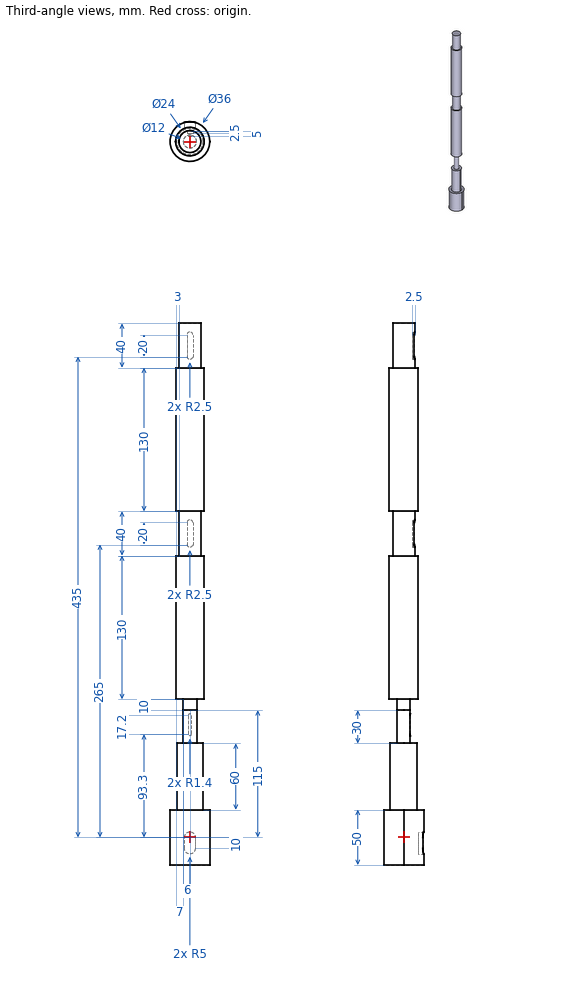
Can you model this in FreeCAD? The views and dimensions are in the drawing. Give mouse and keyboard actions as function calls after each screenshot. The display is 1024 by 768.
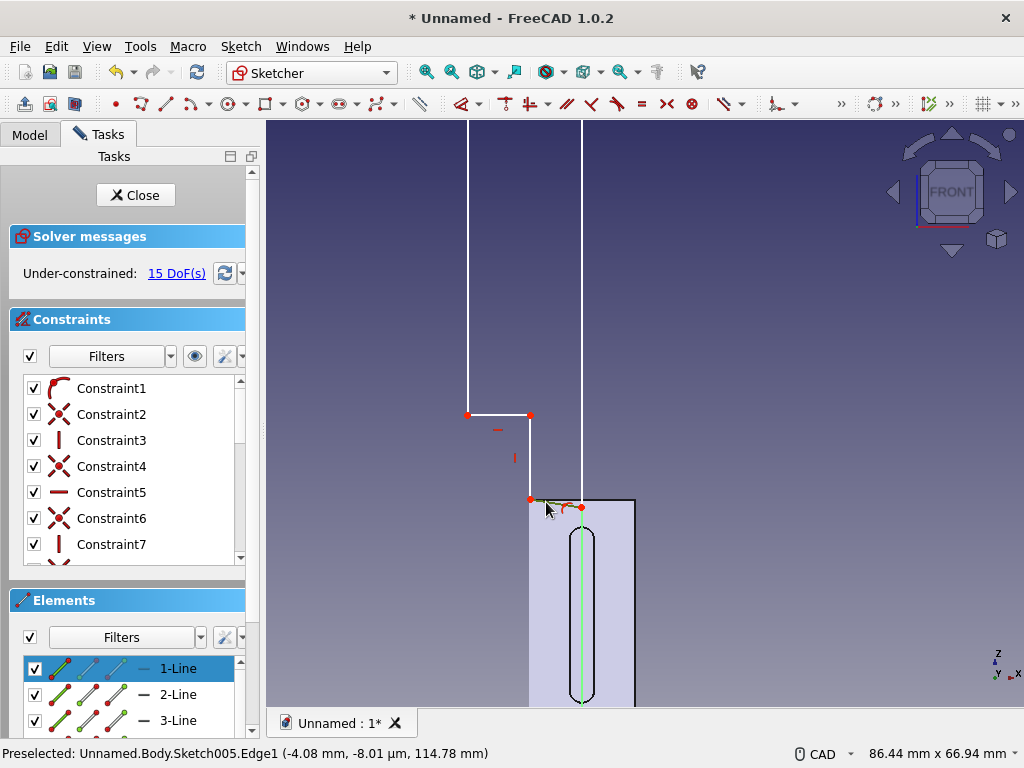
key(h)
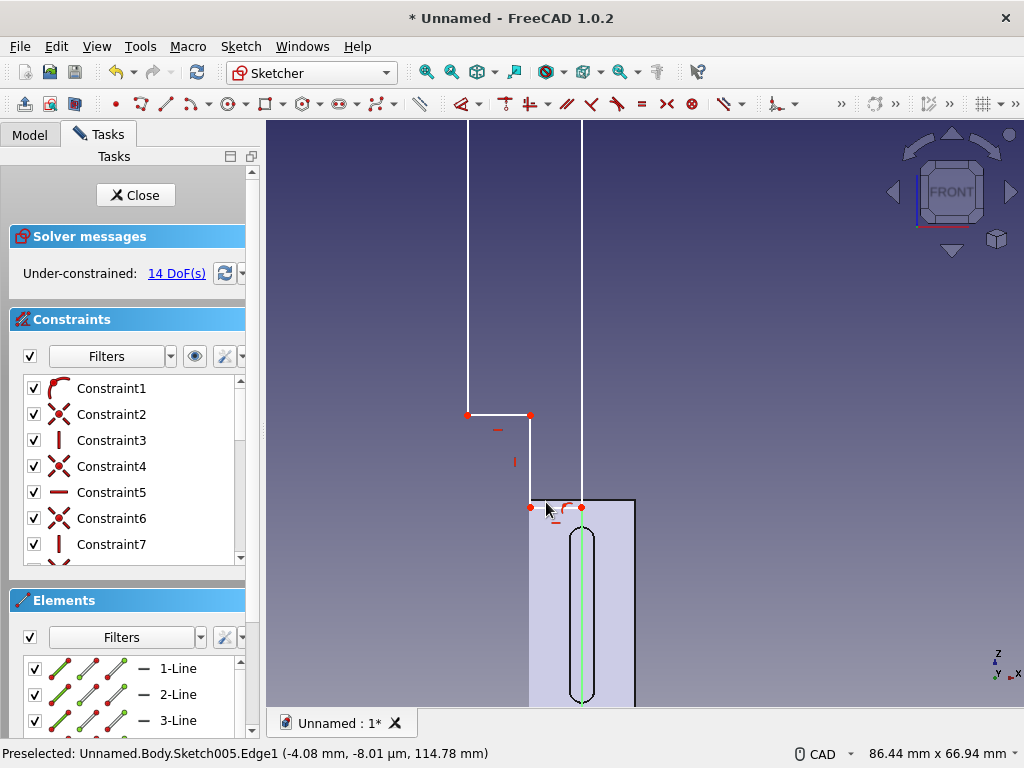
scroll(582, 508, down, 12)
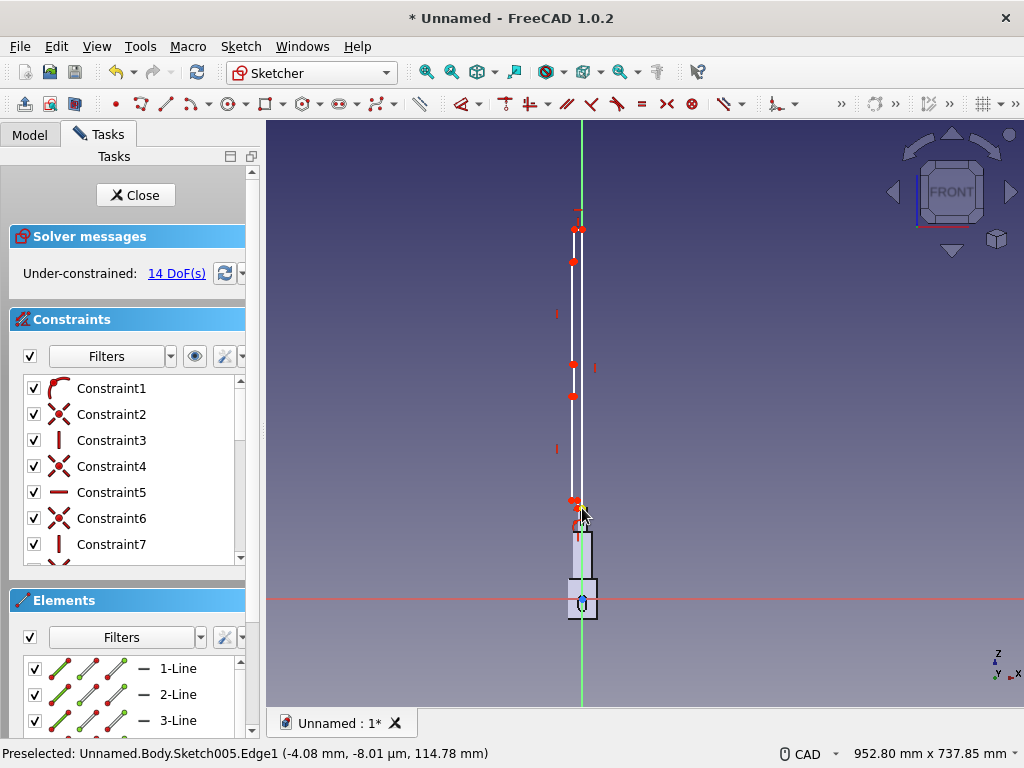
scroll(573, 397, up, 14)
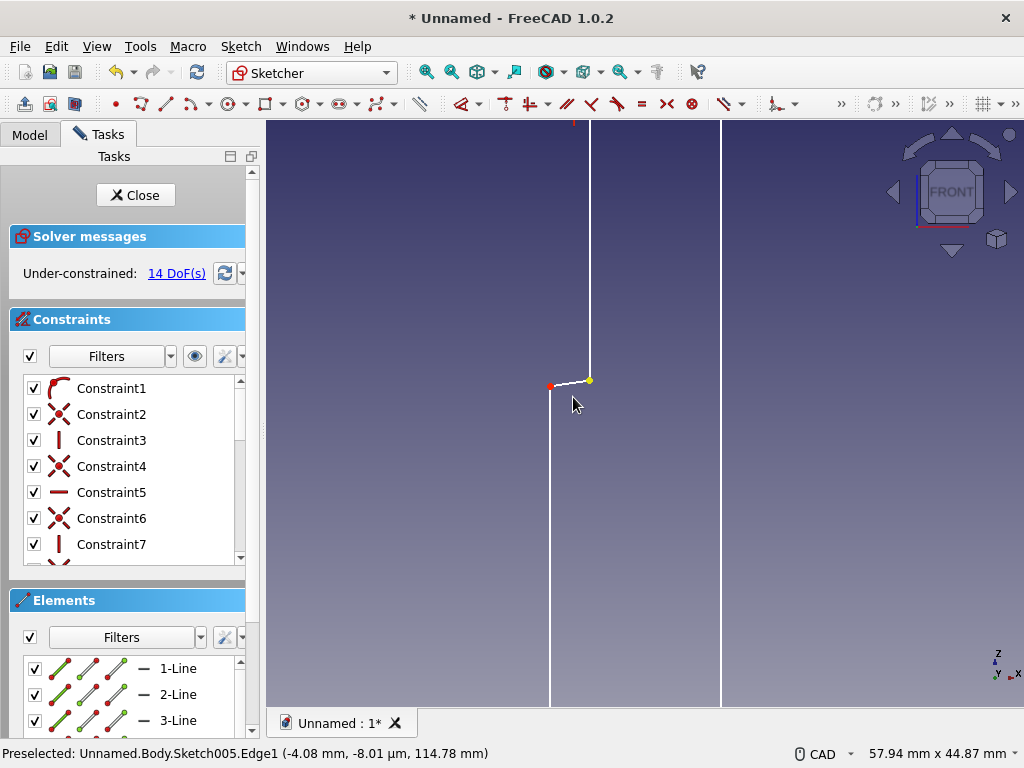
click(566, 384)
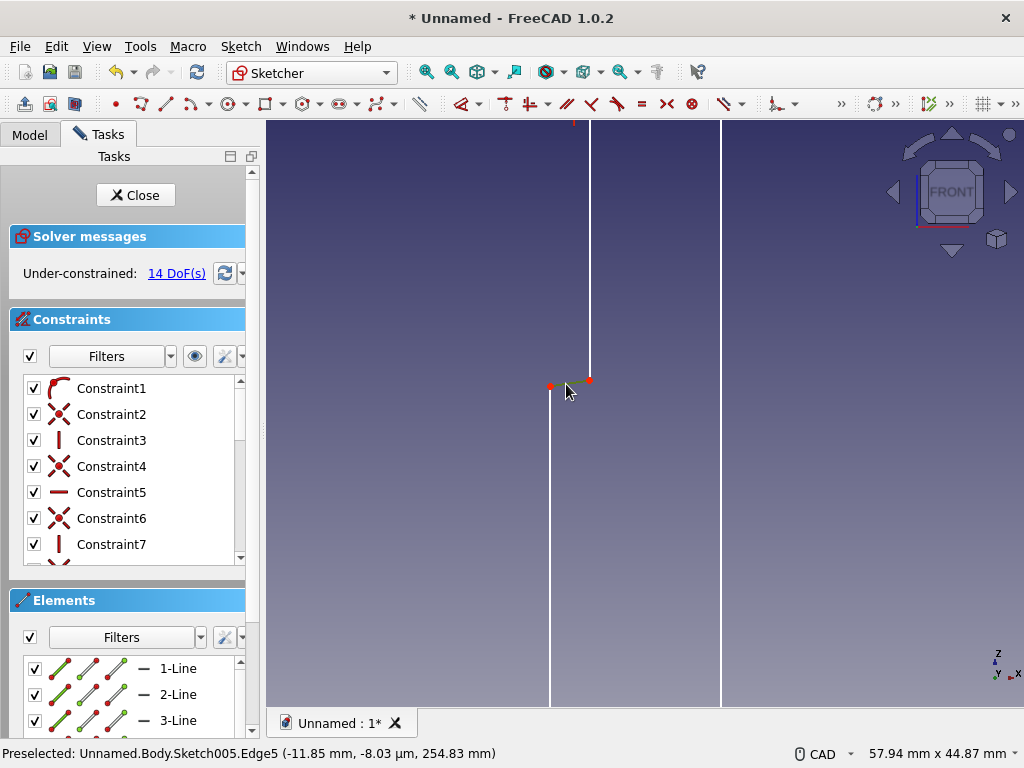
click(548, 104)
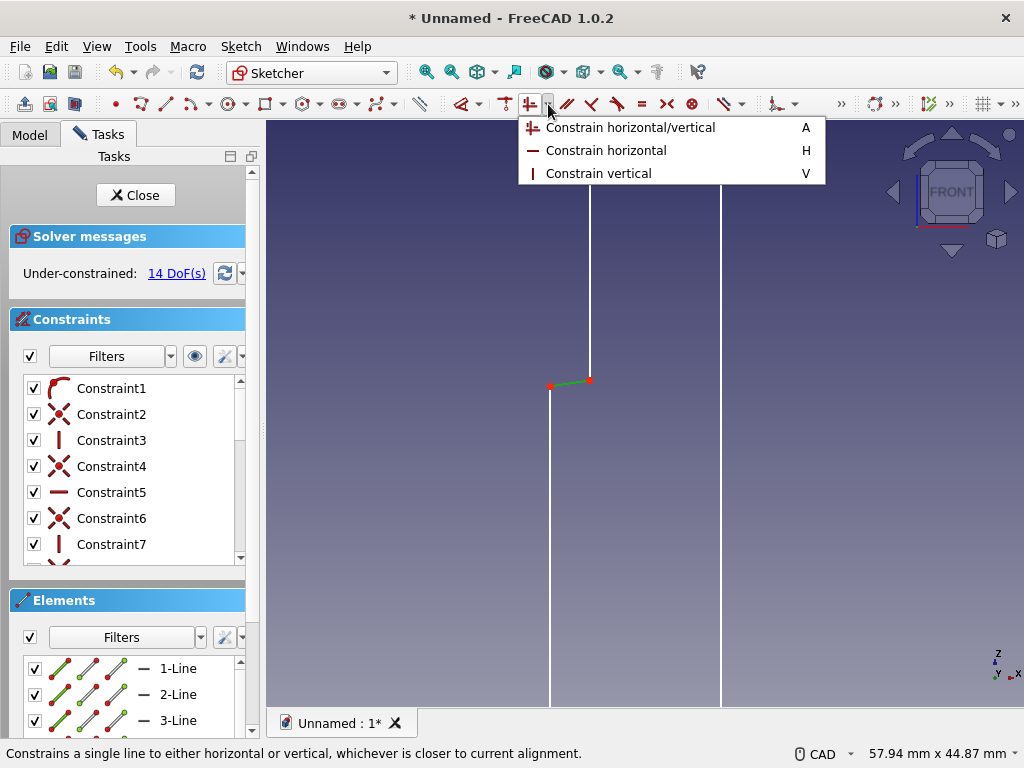
click(672, 150)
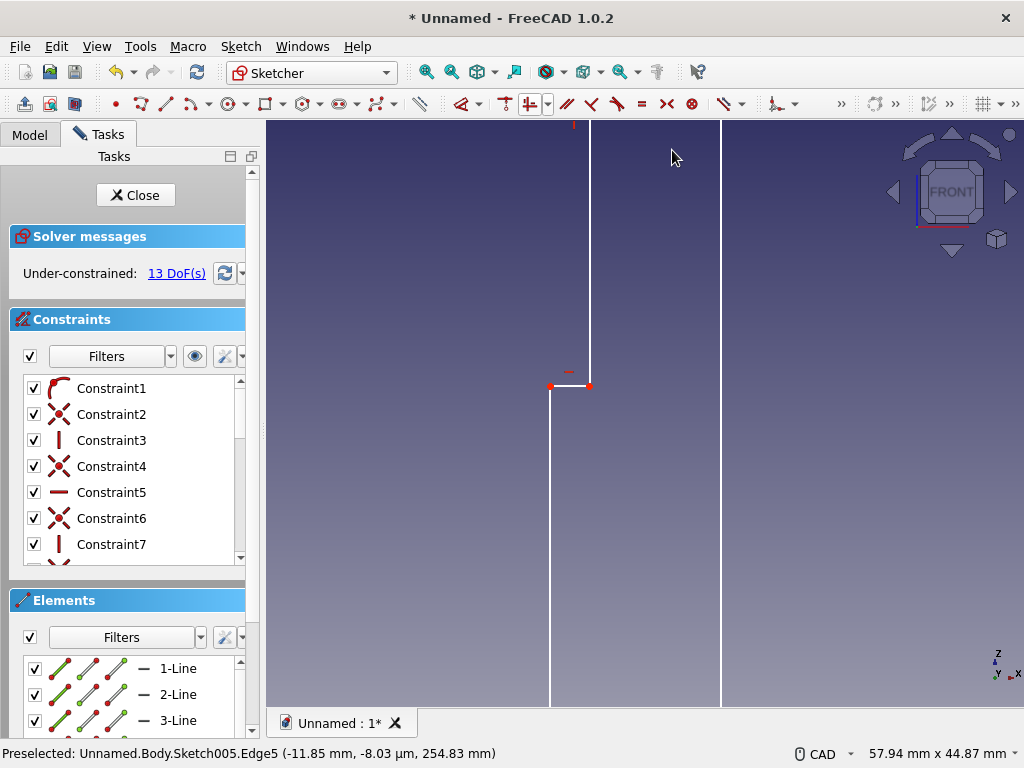
scroll(573, 396, down, 14)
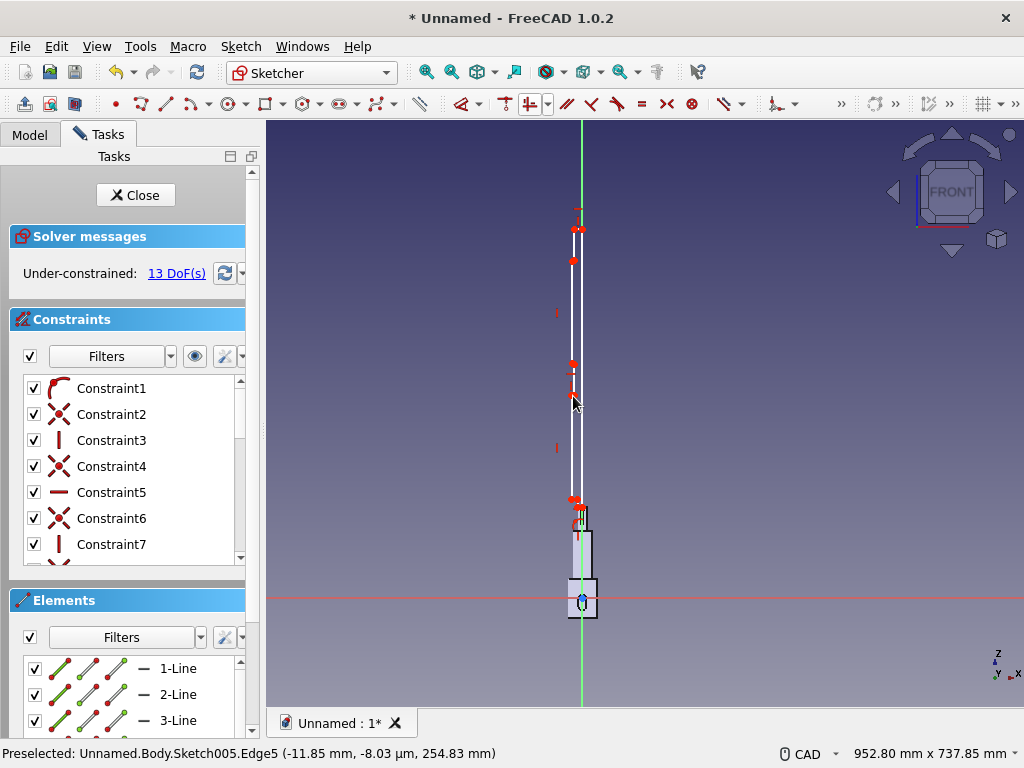
scroll(574, 364, up, 14)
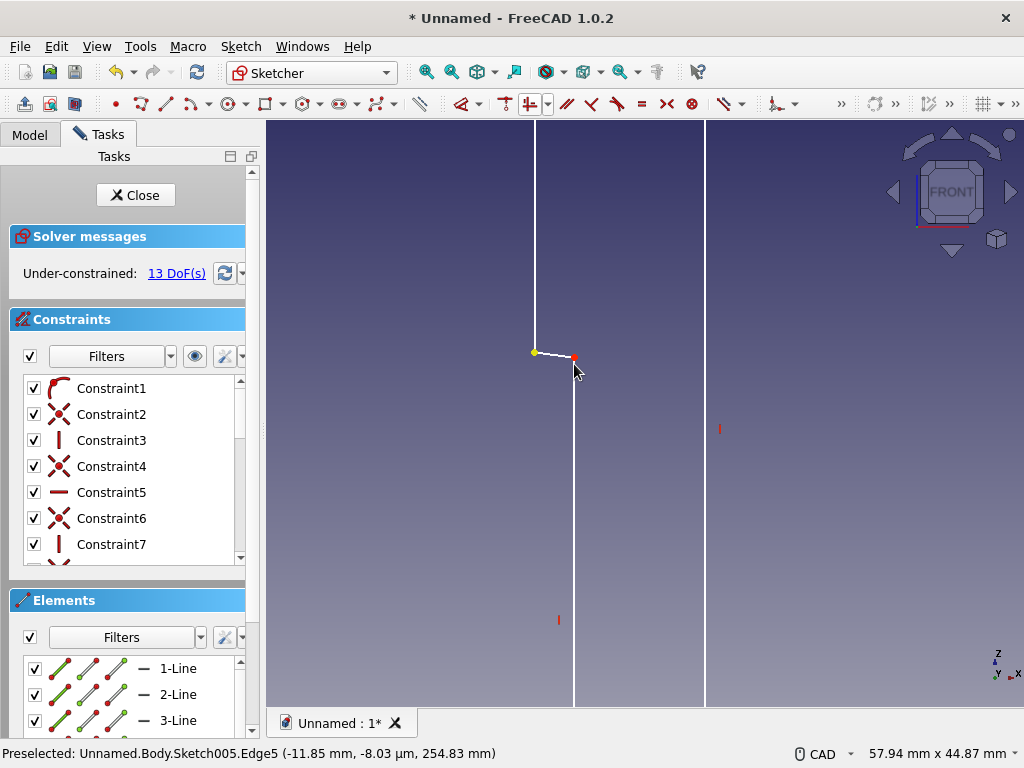
click(562, 356)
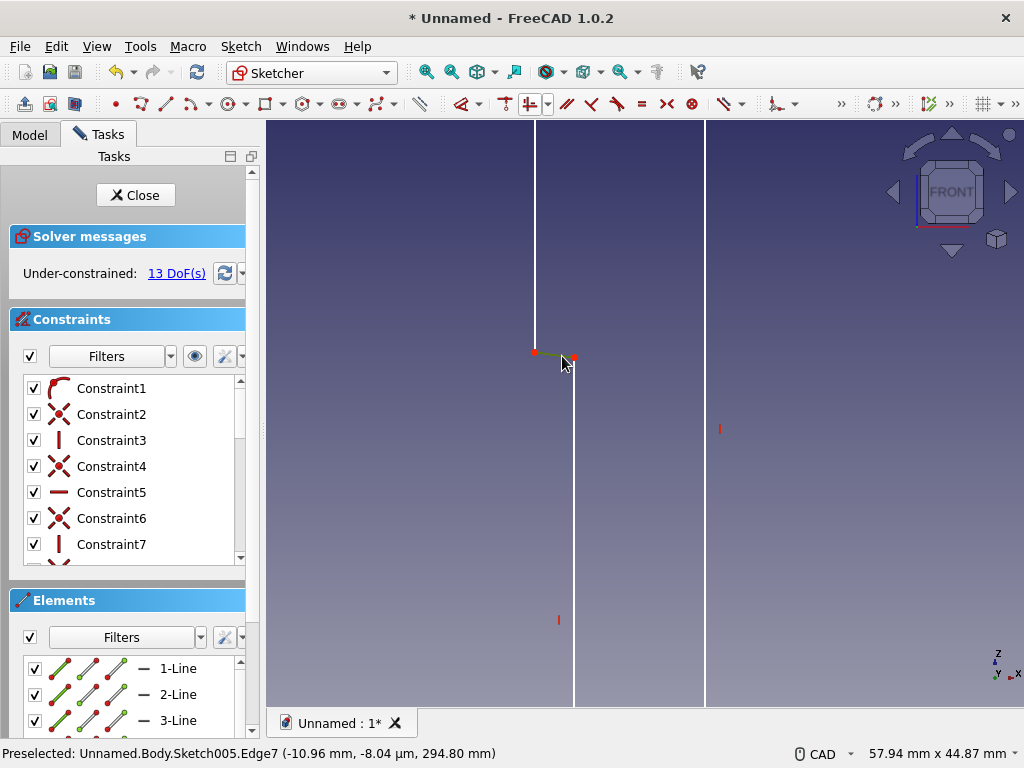
key(h)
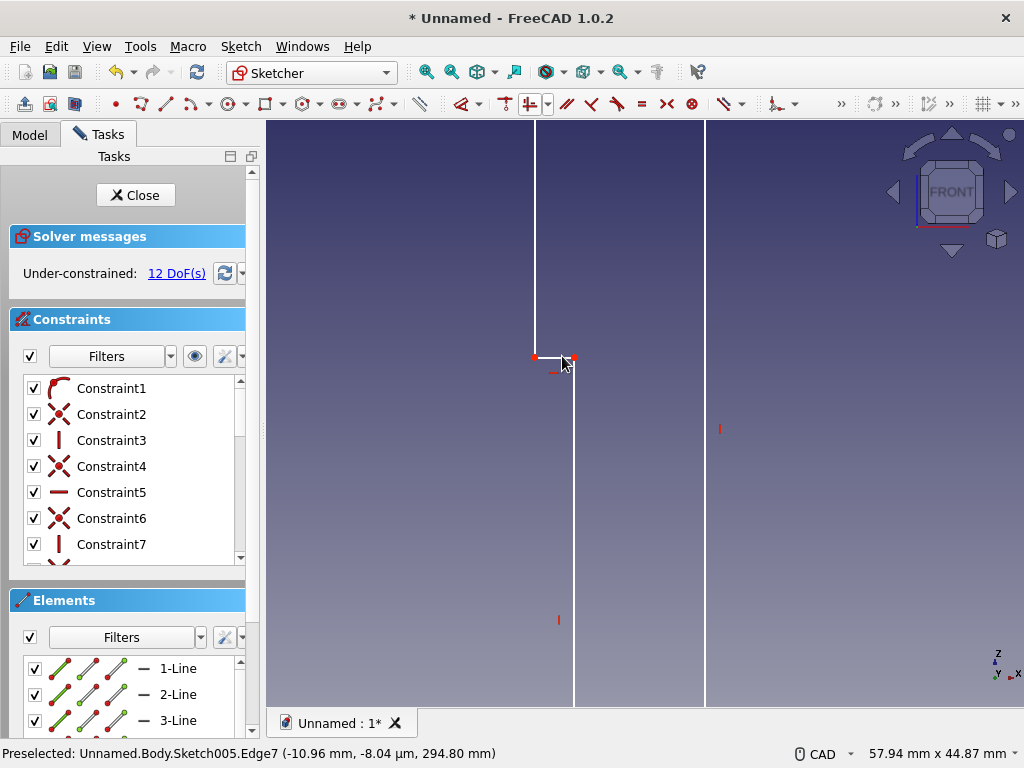
scroll(574, 364, down, 14)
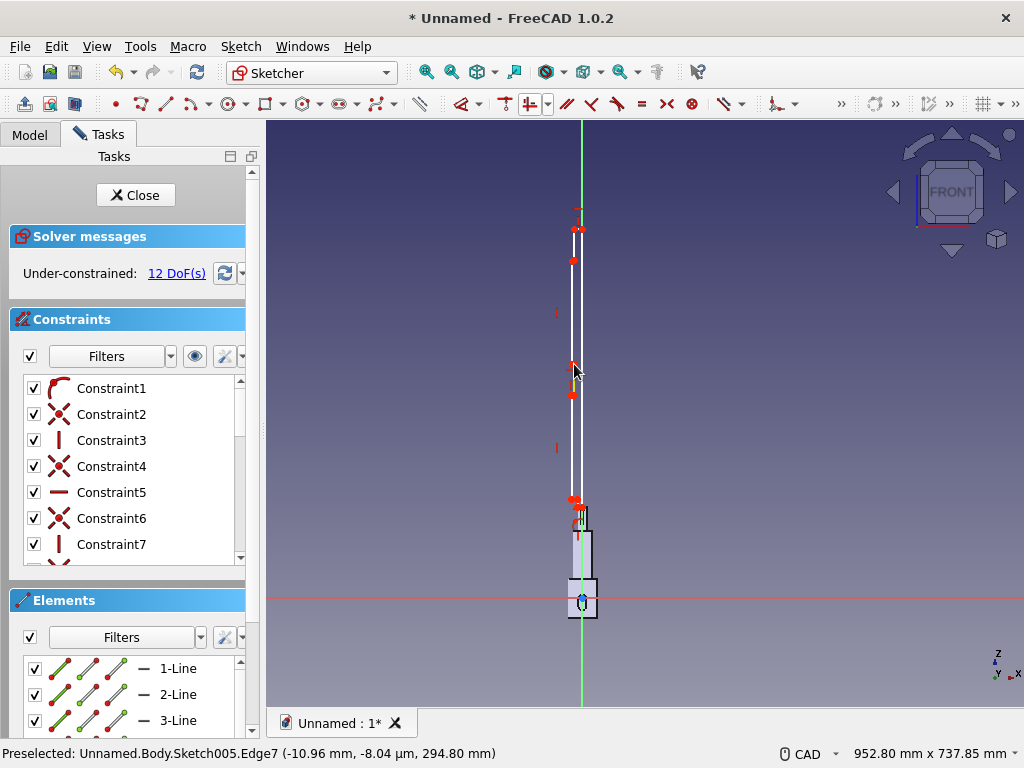
scroll(573, 261, up, 14)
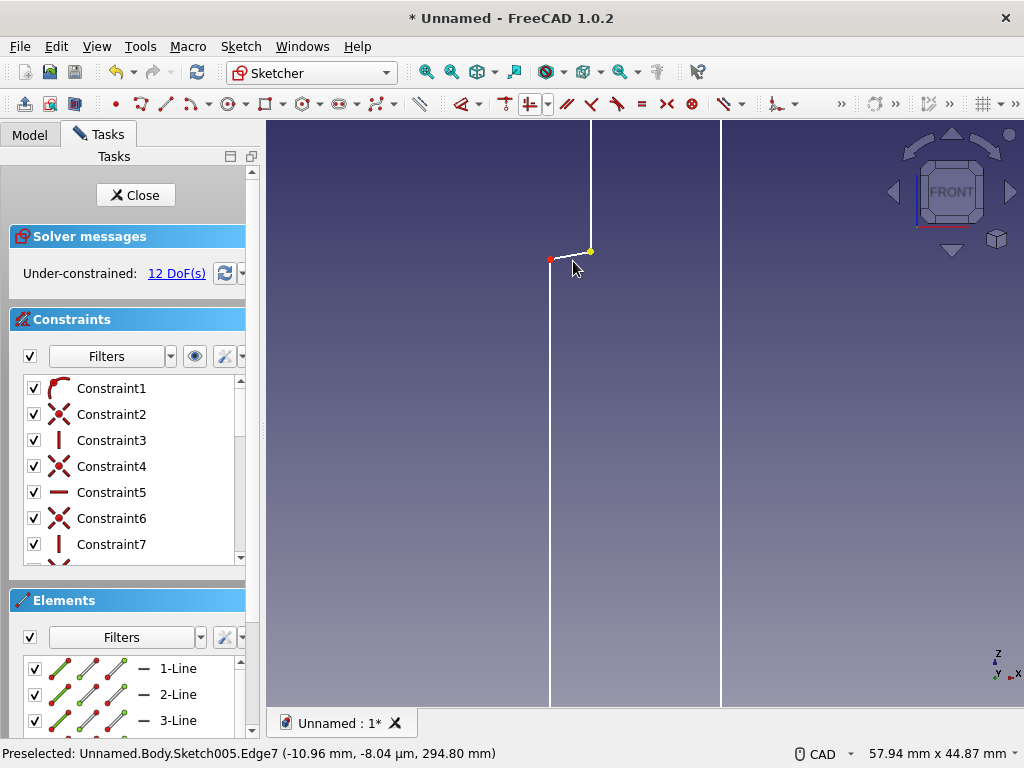
click(563, 257)